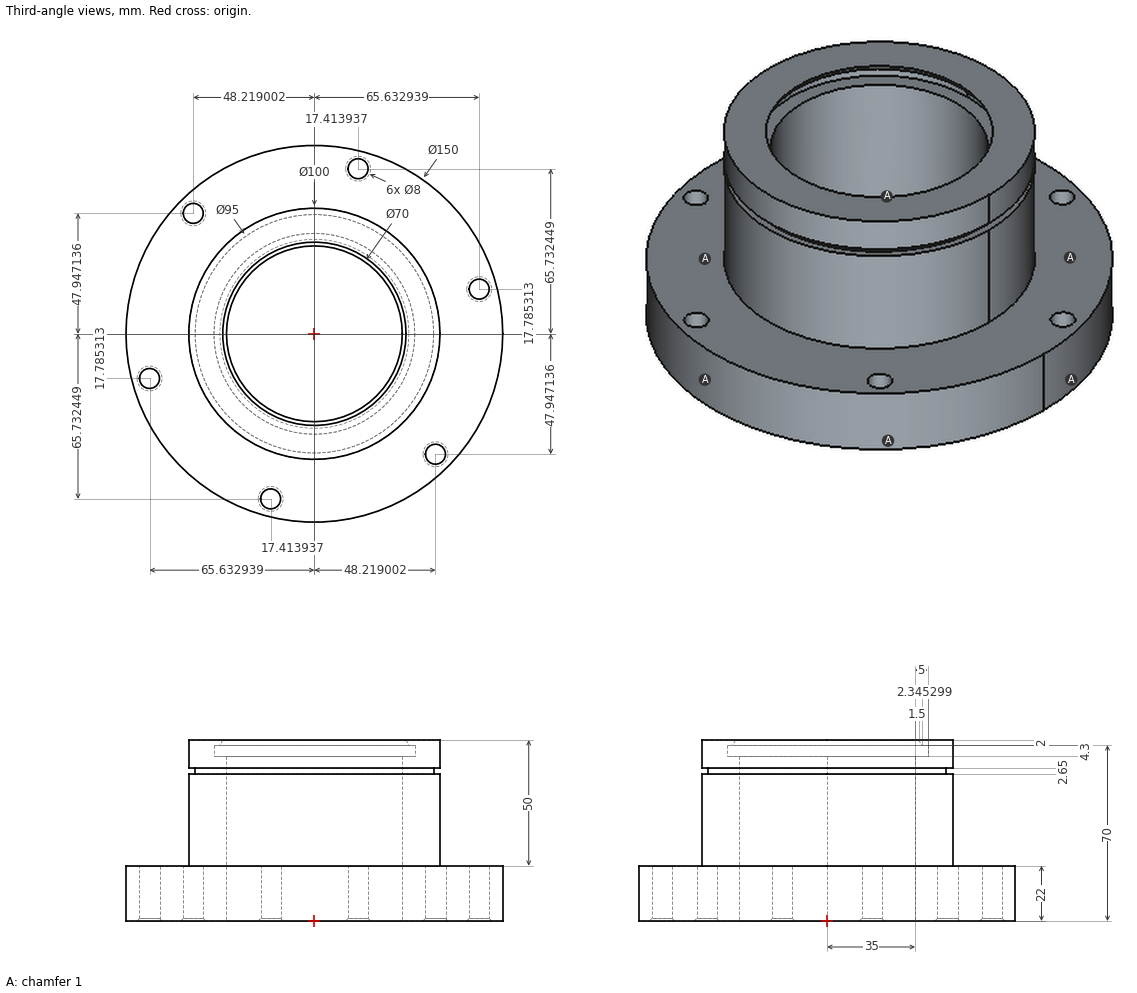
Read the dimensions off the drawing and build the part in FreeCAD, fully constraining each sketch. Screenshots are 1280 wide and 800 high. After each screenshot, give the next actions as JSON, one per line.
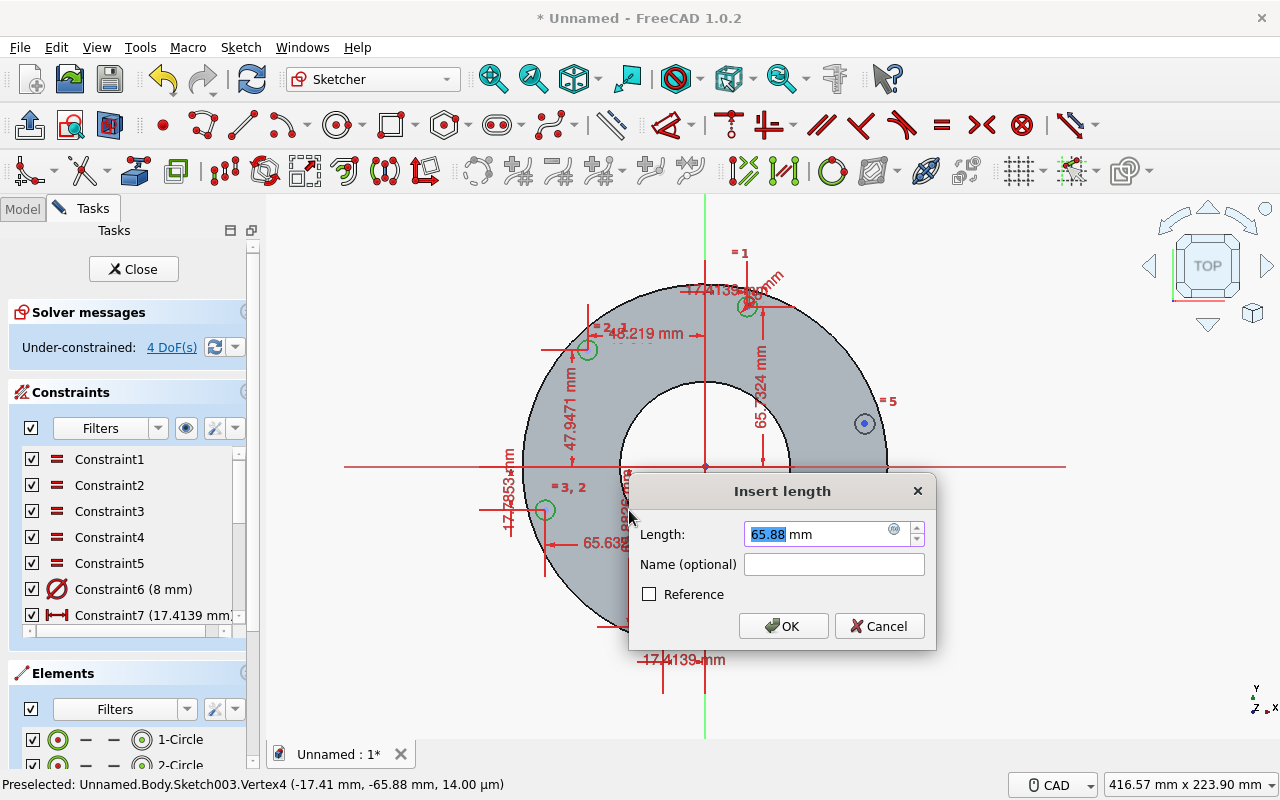
{"action": "type", "text": "65.732449"}
{"action": "key", "text": "Return"}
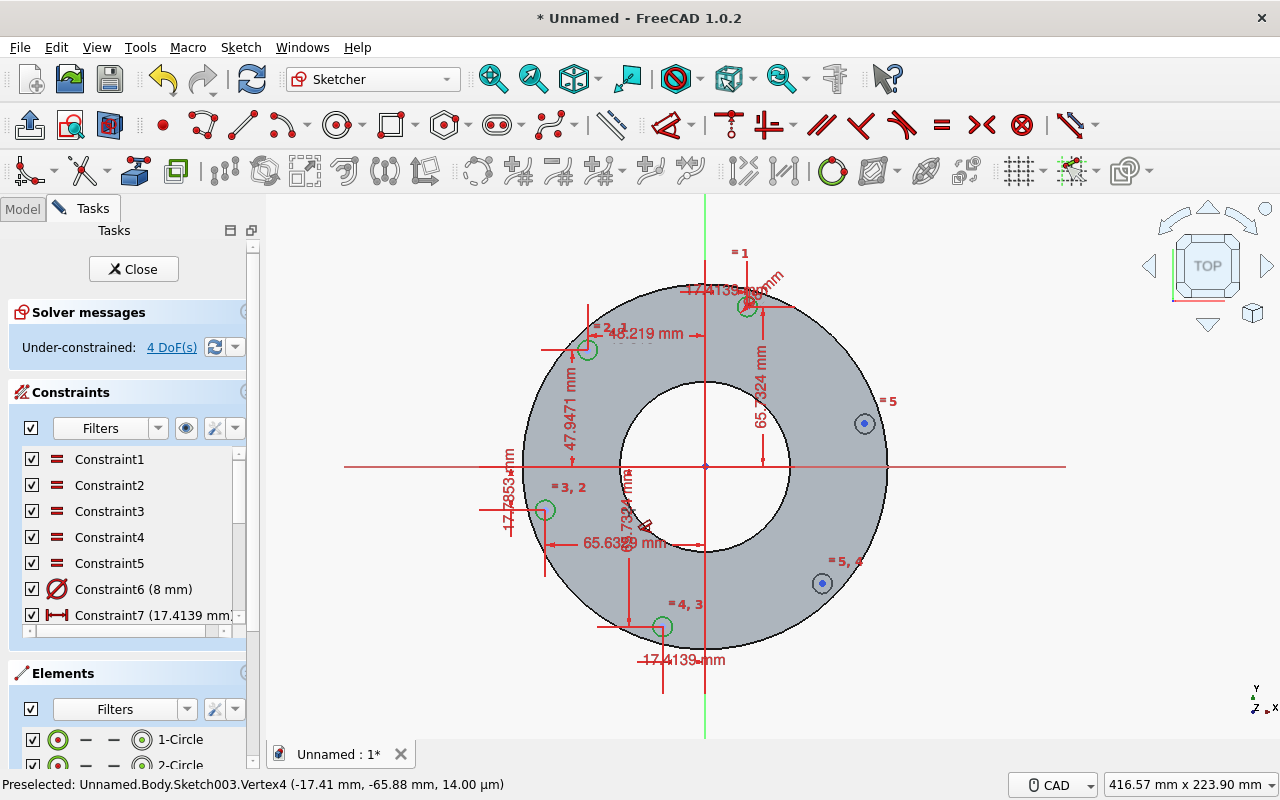
{"action": "left_click", "coordinate": [822, 584]}
{"action": "left_click", "coordinate": [764, 618]}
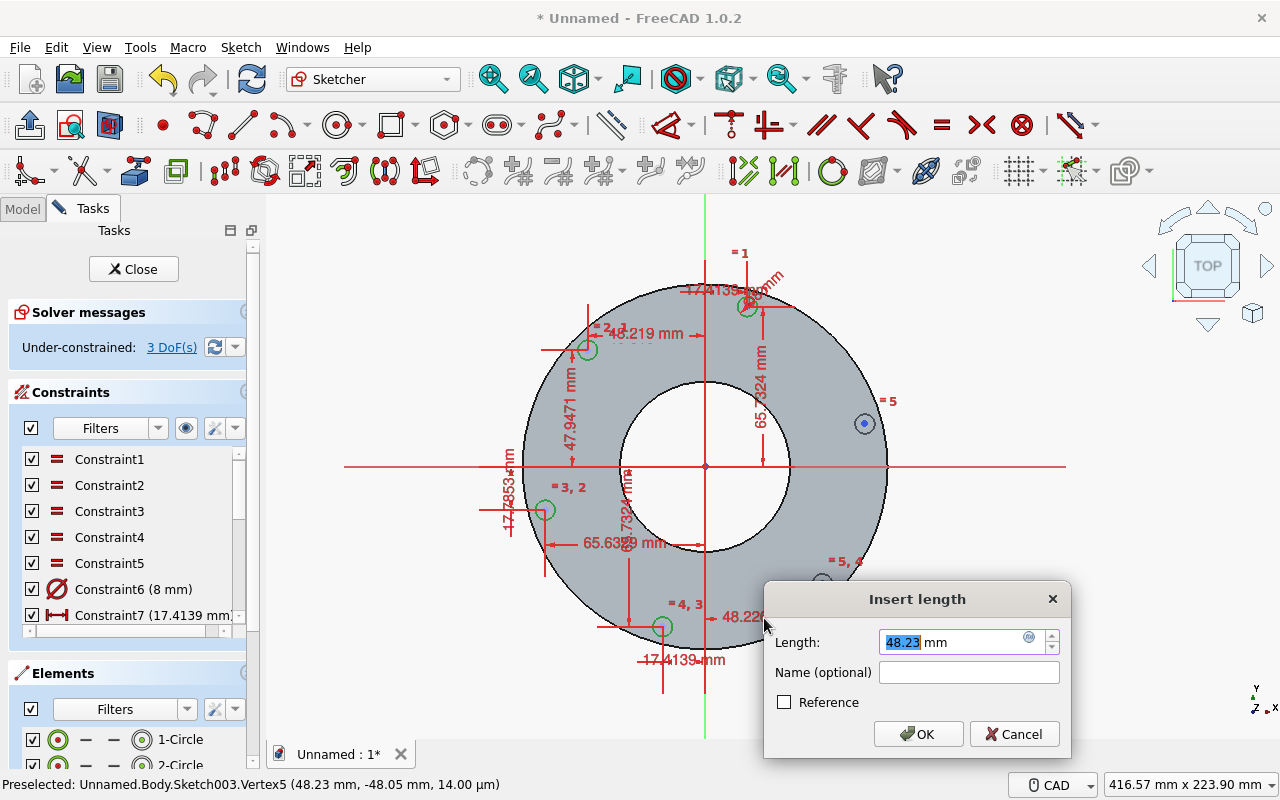
{"action": "type", "text": "48.219002"}
{"action": "key", "text": "Return"}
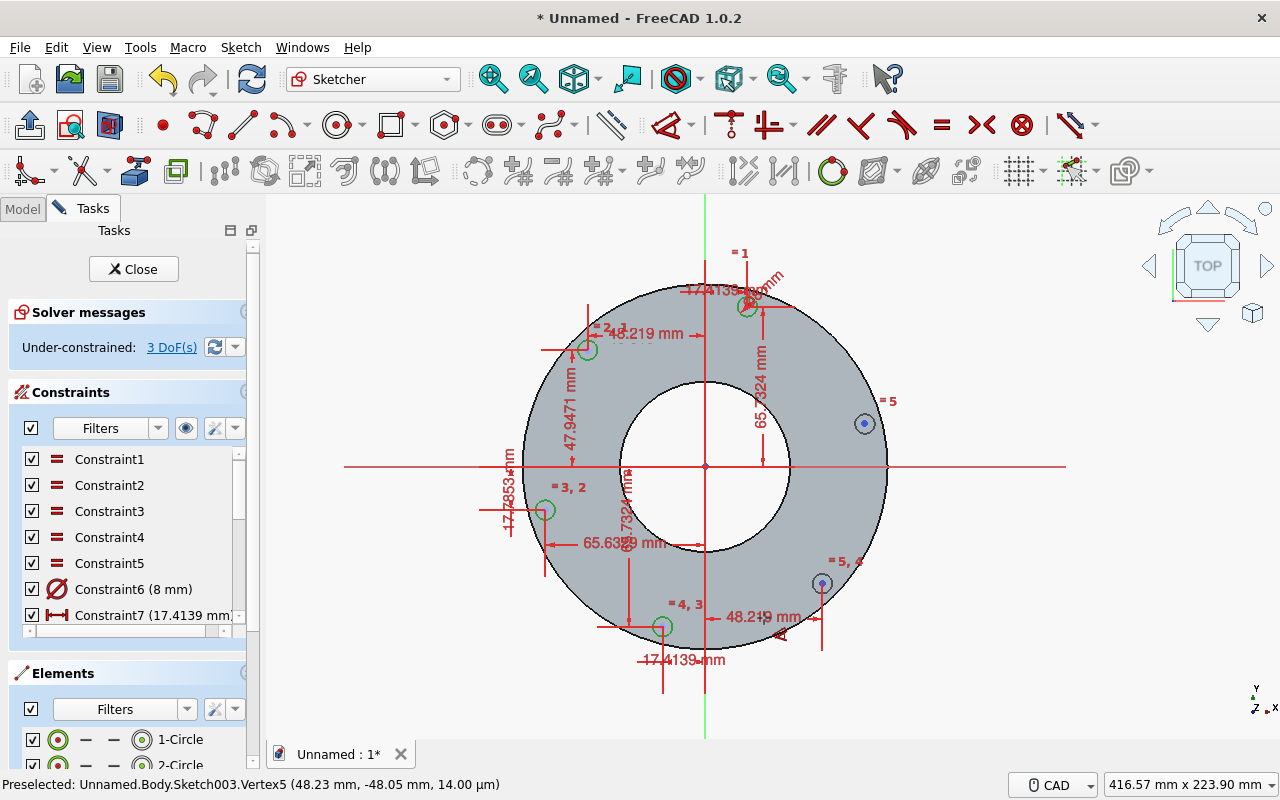
{"action": "left_click", "coordinate": [822, 584]}
{"action": "left_click", "coordinate": [856, 525]}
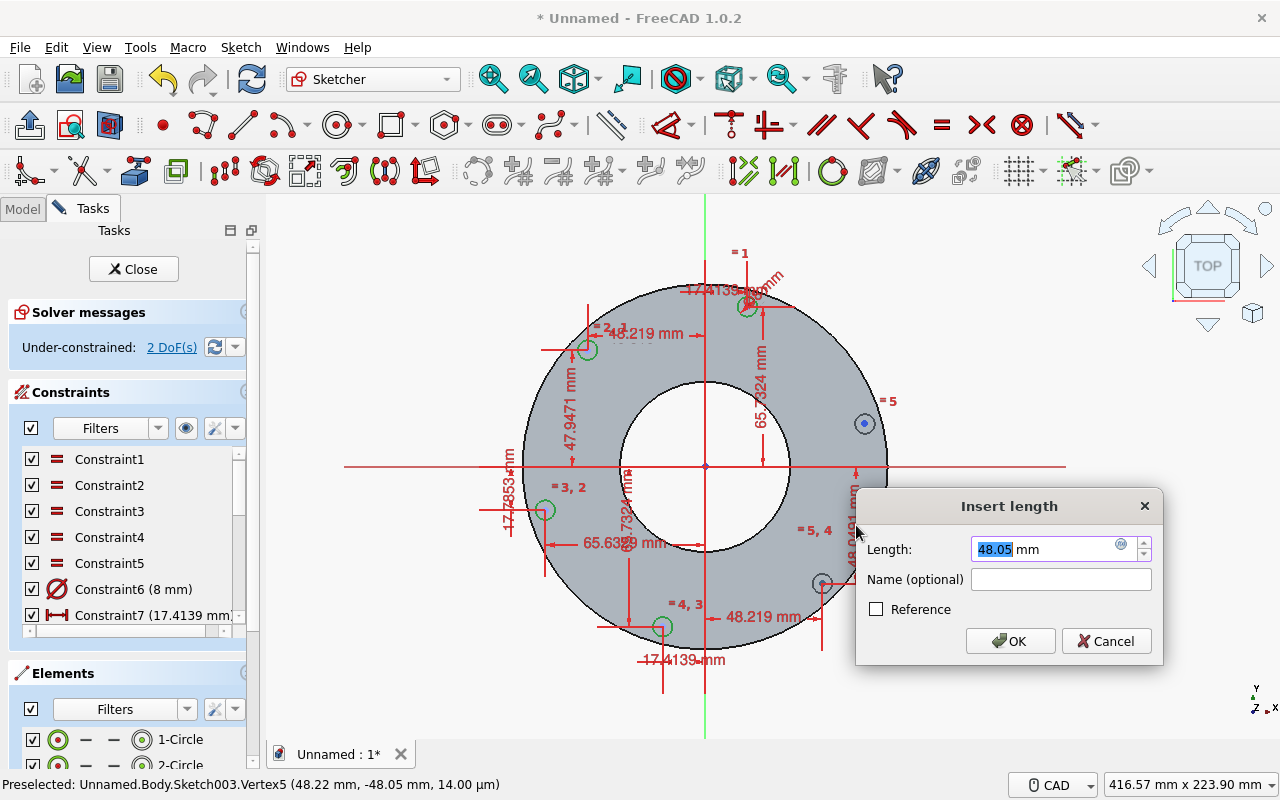
{"action": "type", "text": "47.947136"}
{"action": "key", "text": "Return"}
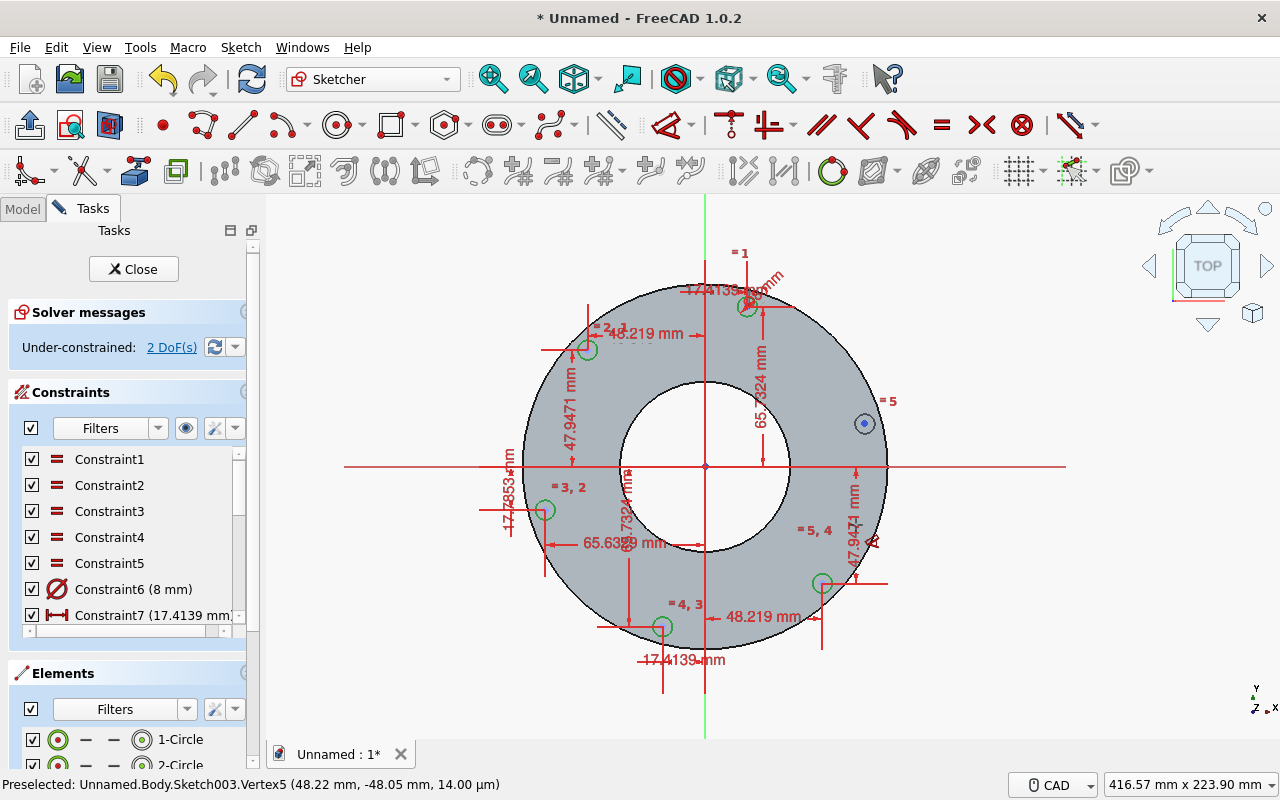
{"action": "left_click", "coordinate": [865, 424]}
{"action": "left_click", "coordinate": [841, 390]}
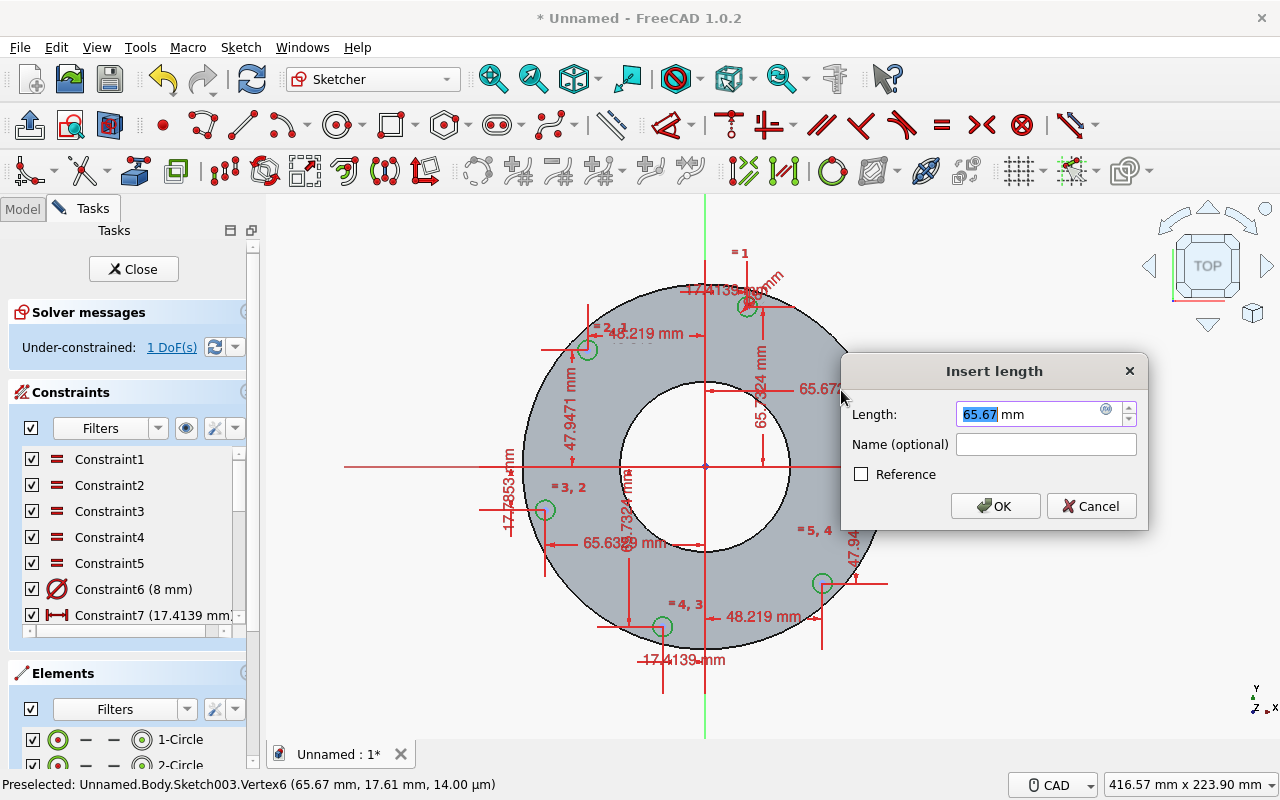
{"action": "type", "text": "65.632939"}
{"action": "key", "text": "Return"}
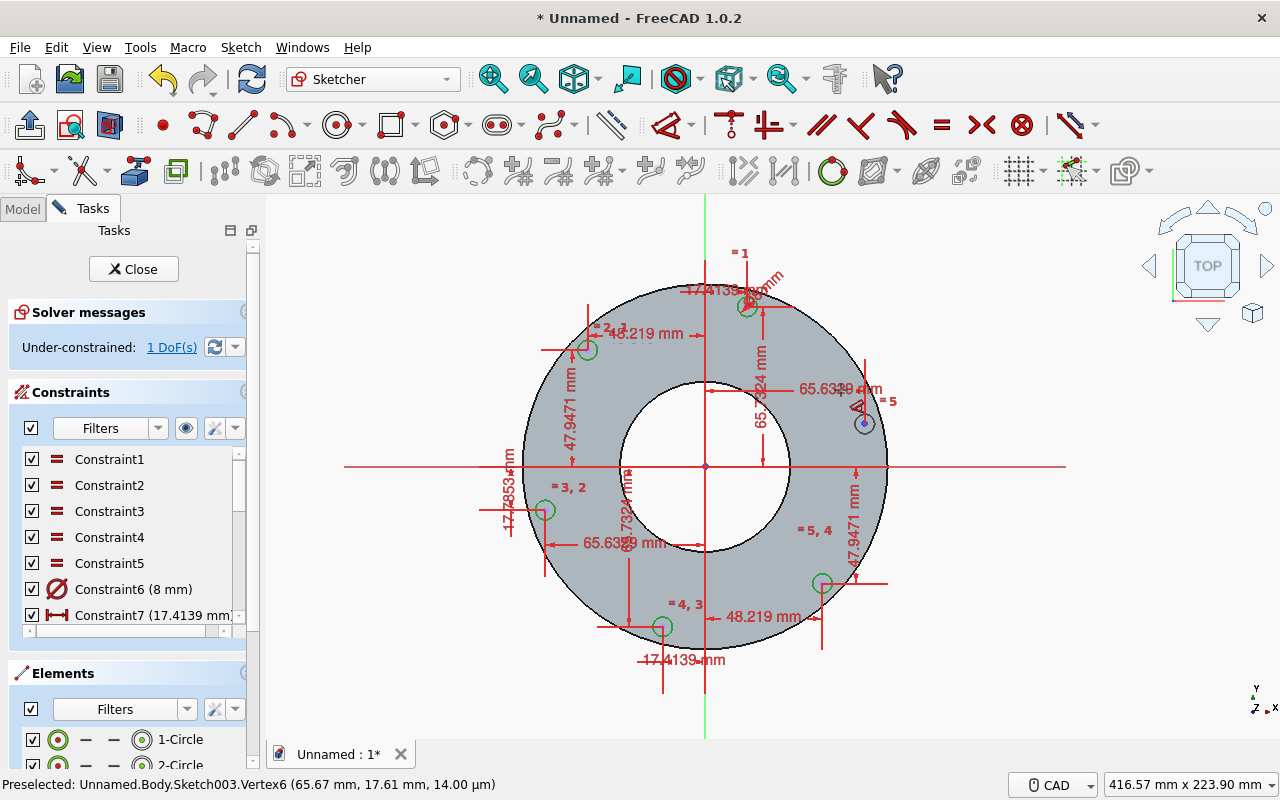
{"action": "left_click", "coordinate": [865, 424]}
{"action": "left_click", "coordinate": [899, 445]}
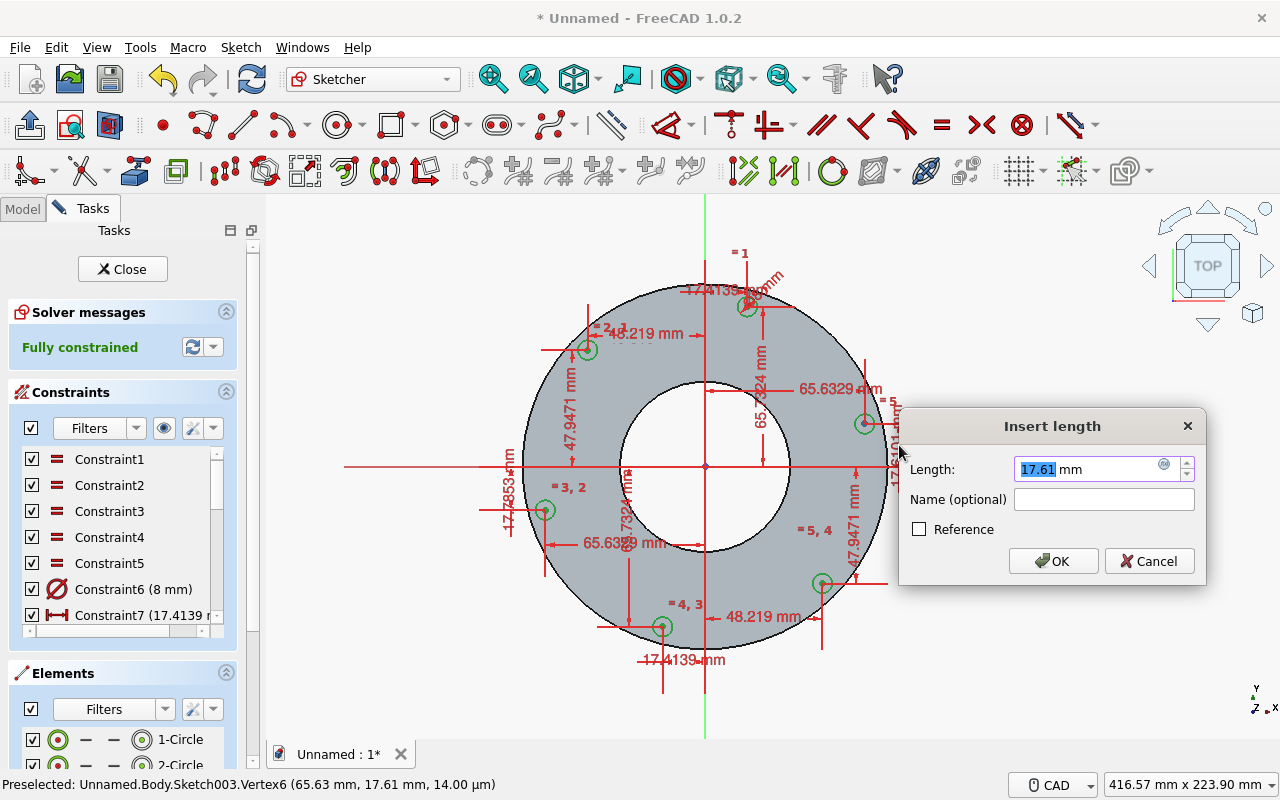
{"action": "type", "text": "17.785313"}
{"action": "key", "text": "Return"}
{"action": "key", "text": "Escape"}